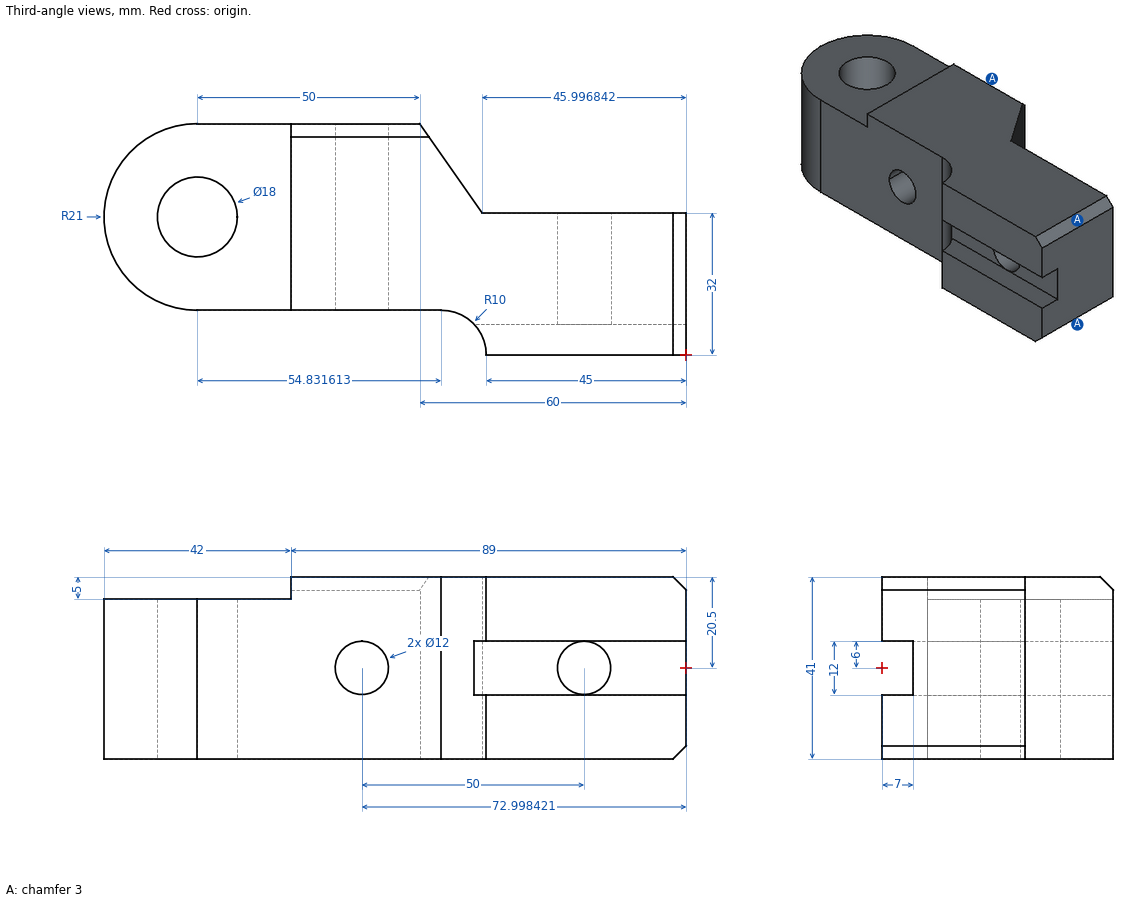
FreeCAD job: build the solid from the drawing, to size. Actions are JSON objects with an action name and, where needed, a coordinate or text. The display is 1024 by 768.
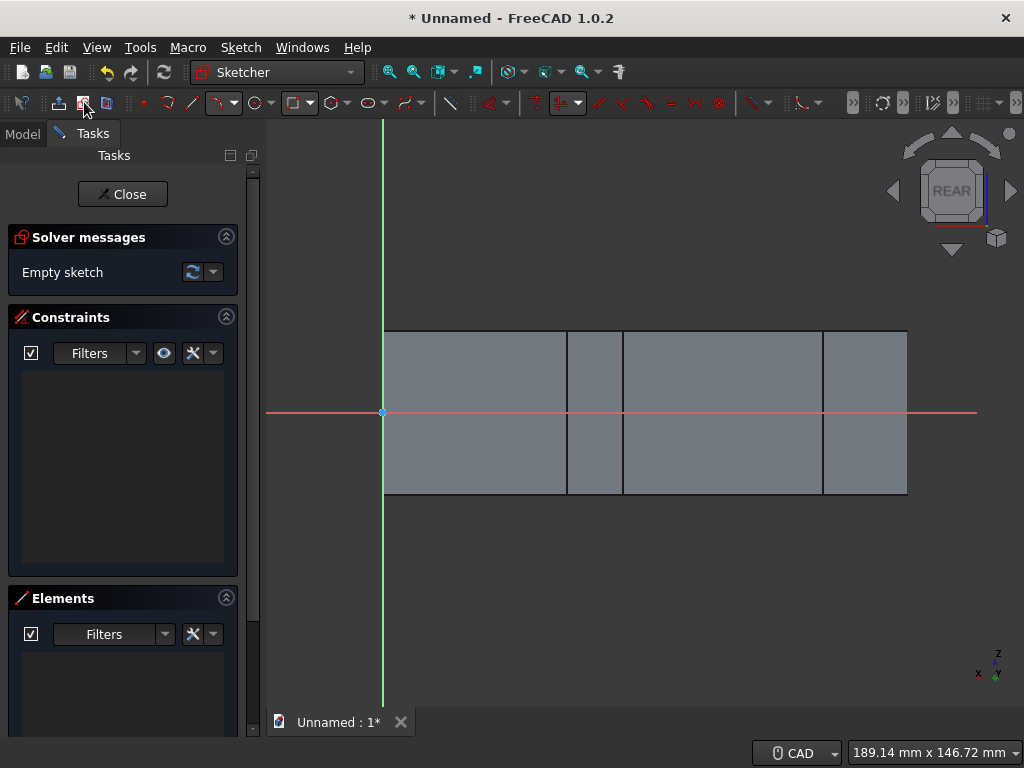
{"action": "scroll", "coordinate": [294, 544], "scroll_direction": "down", "scroll_amount": 1}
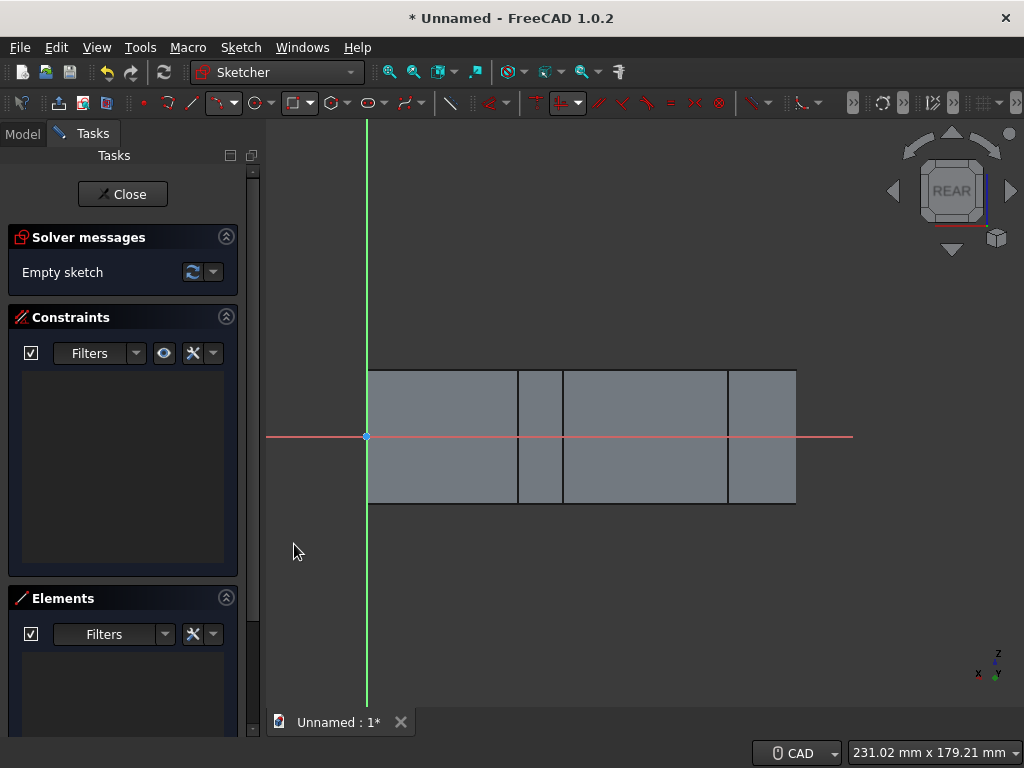
{"action": "left_click", "coordinate": [294, 104]}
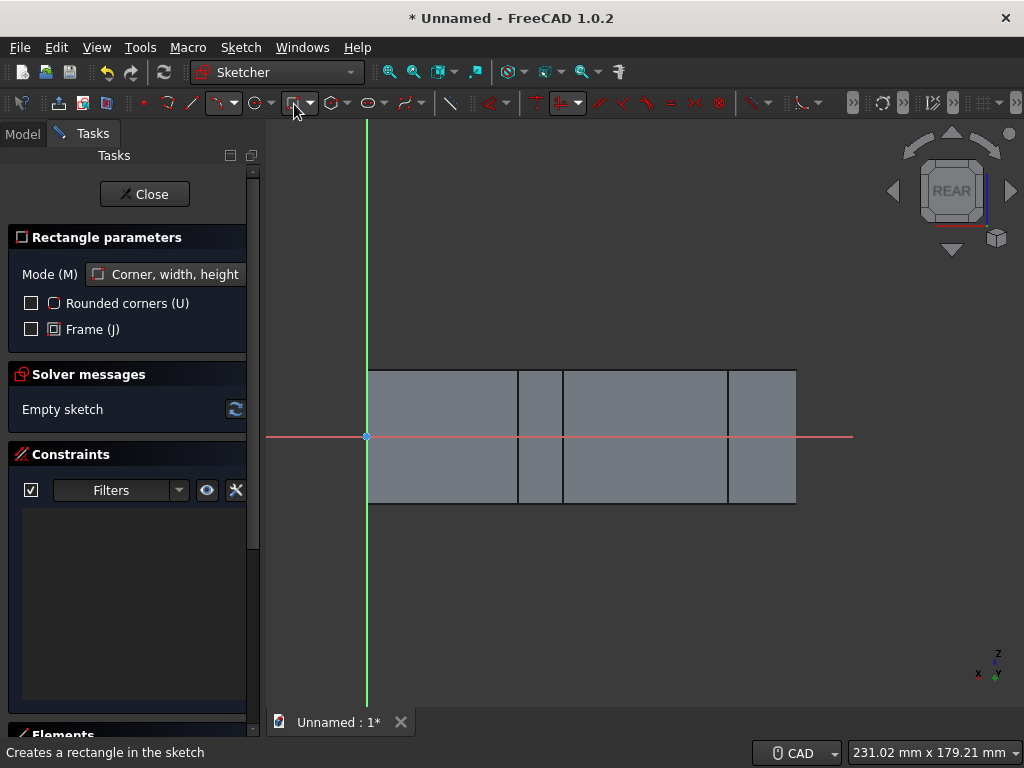
{"action": "left_click", "coordinate": [659, 370]}
{"action": "left_click", "coordinate": [796, 386]}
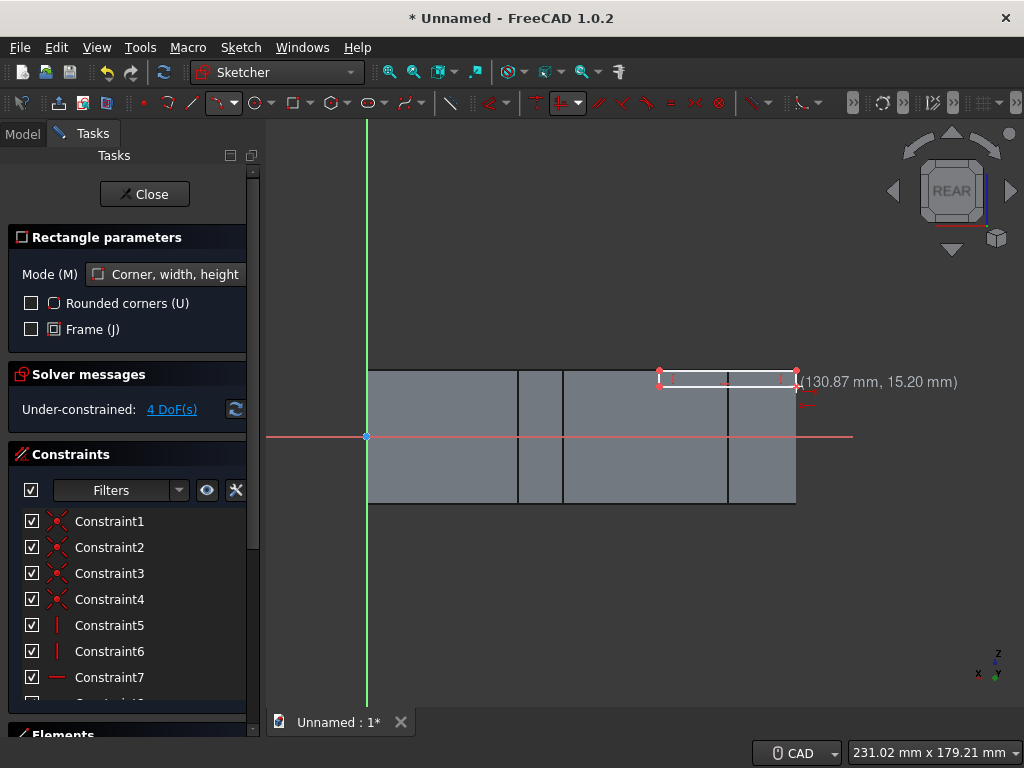
{"action": "left_click", "coordinate": [256, 104]}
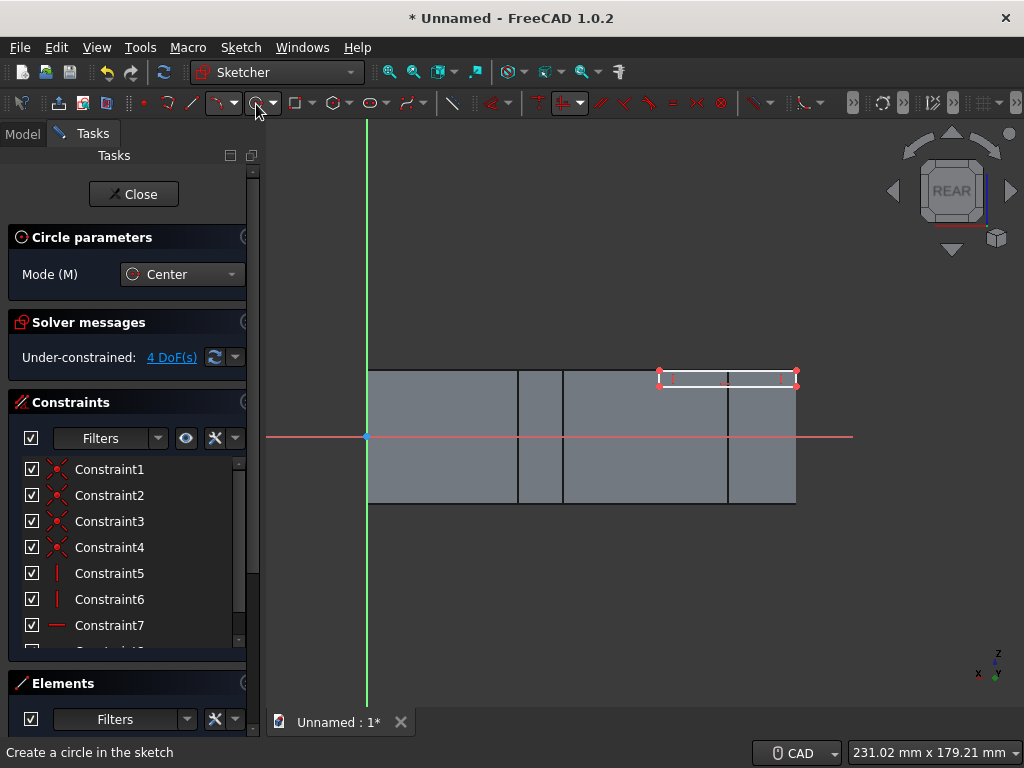
{"action": "left_click", "coordinate": [606, 437]}
{"action": "left_click", "coordinate": [613, 418]}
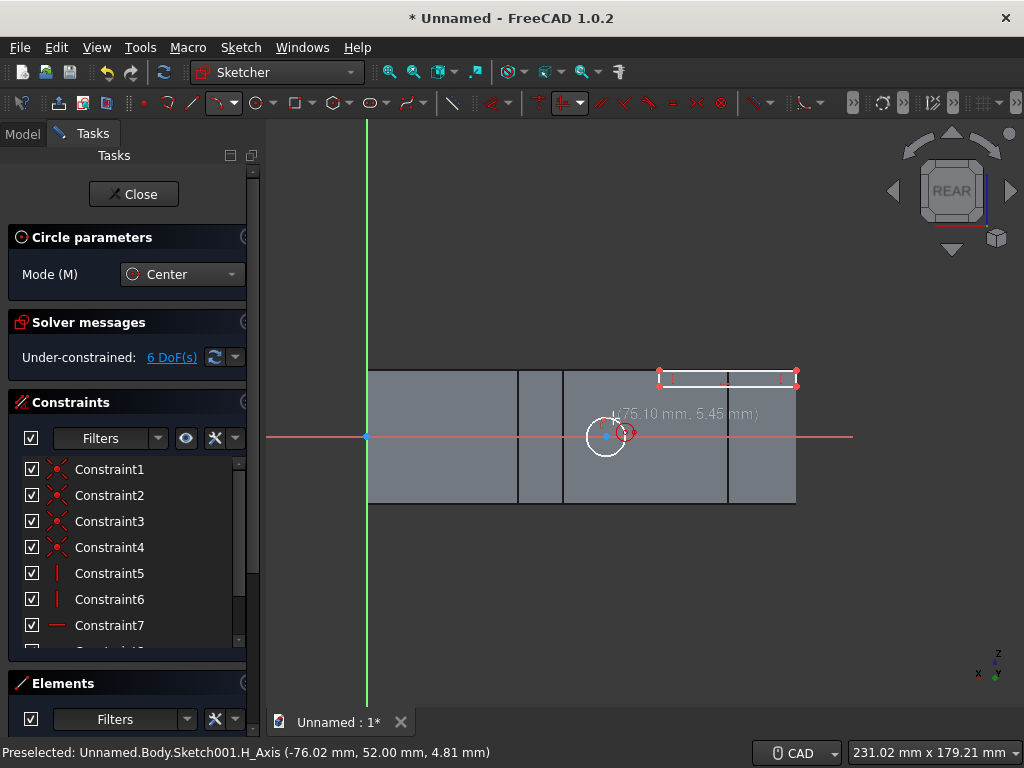
{"action": "left_click", "coordinate": [442, 437]}
{"action": "left_click", "coordinate": [449, 418]}
{"action": "key", "text": "Escape"}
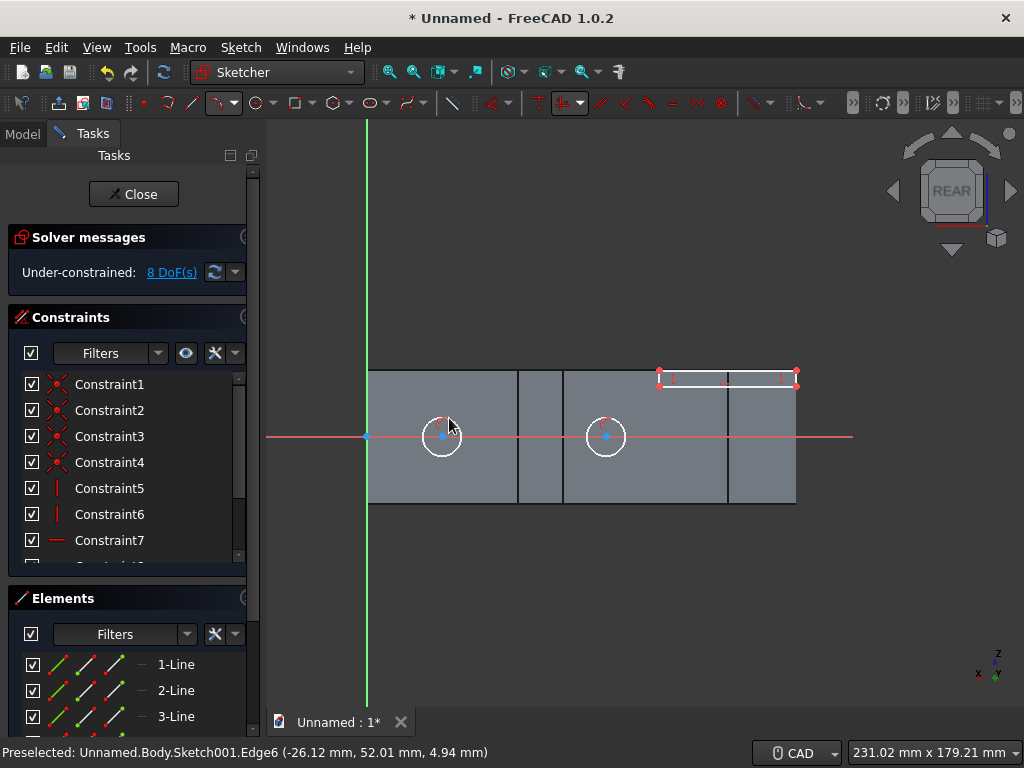
{"action": "left_click", "coordinate": [620, 423]}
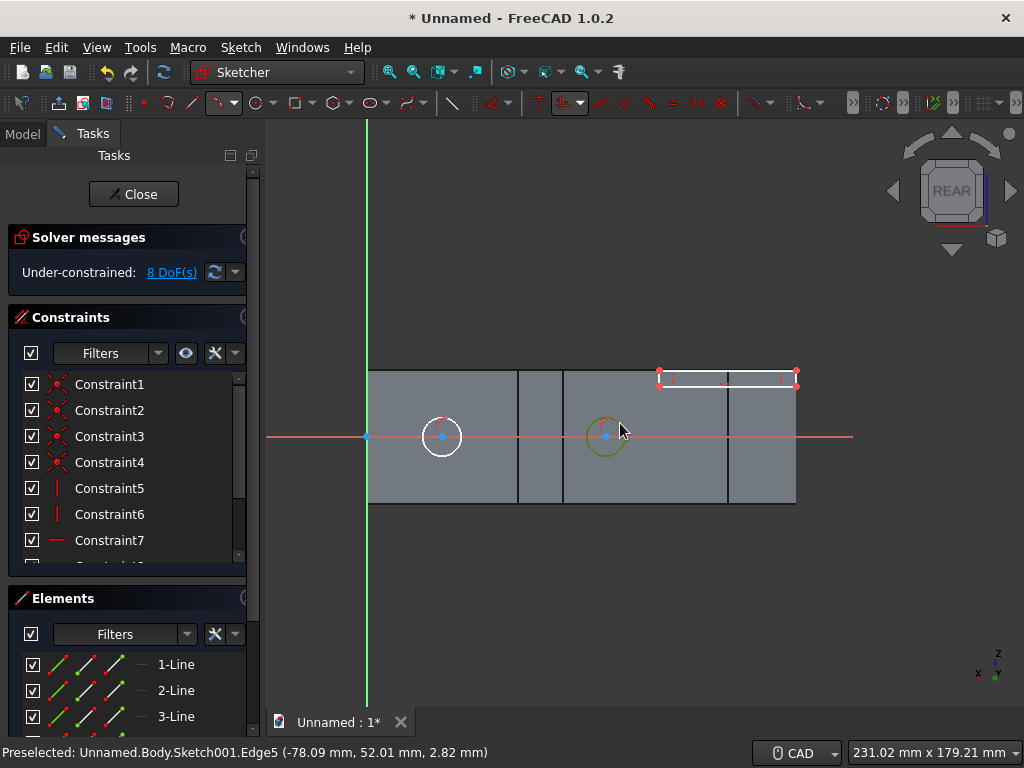
{"action": "left_click", "coordinate": [456, 423]}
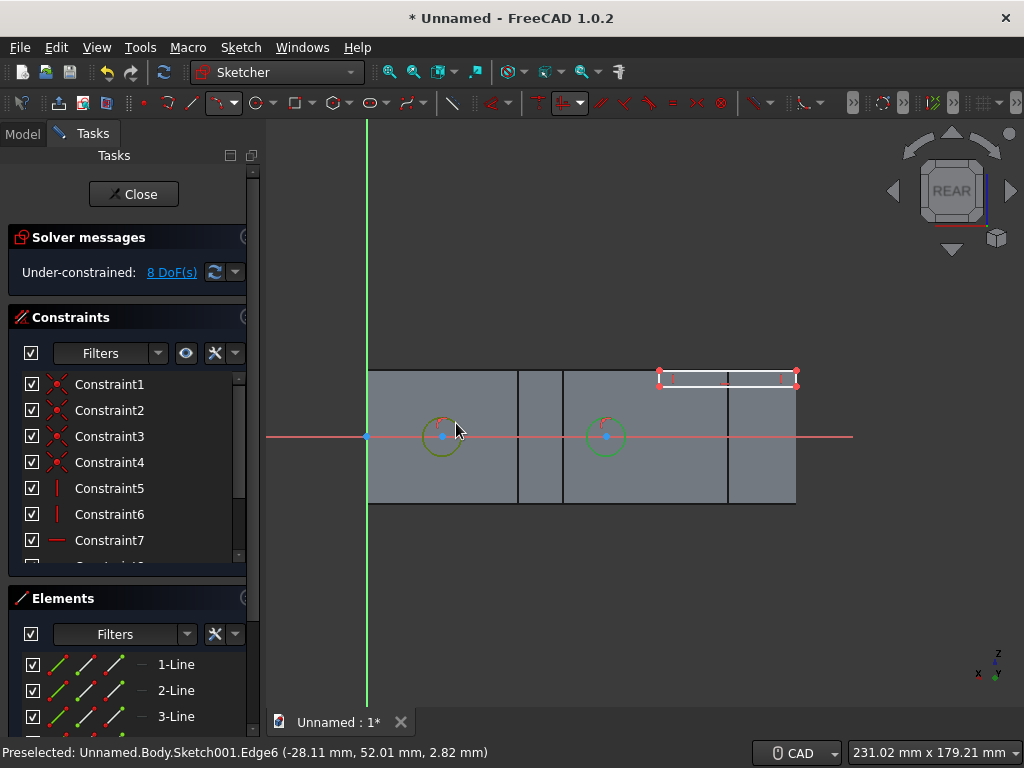
{"action": "left_click", "coordinate": [674, 104]}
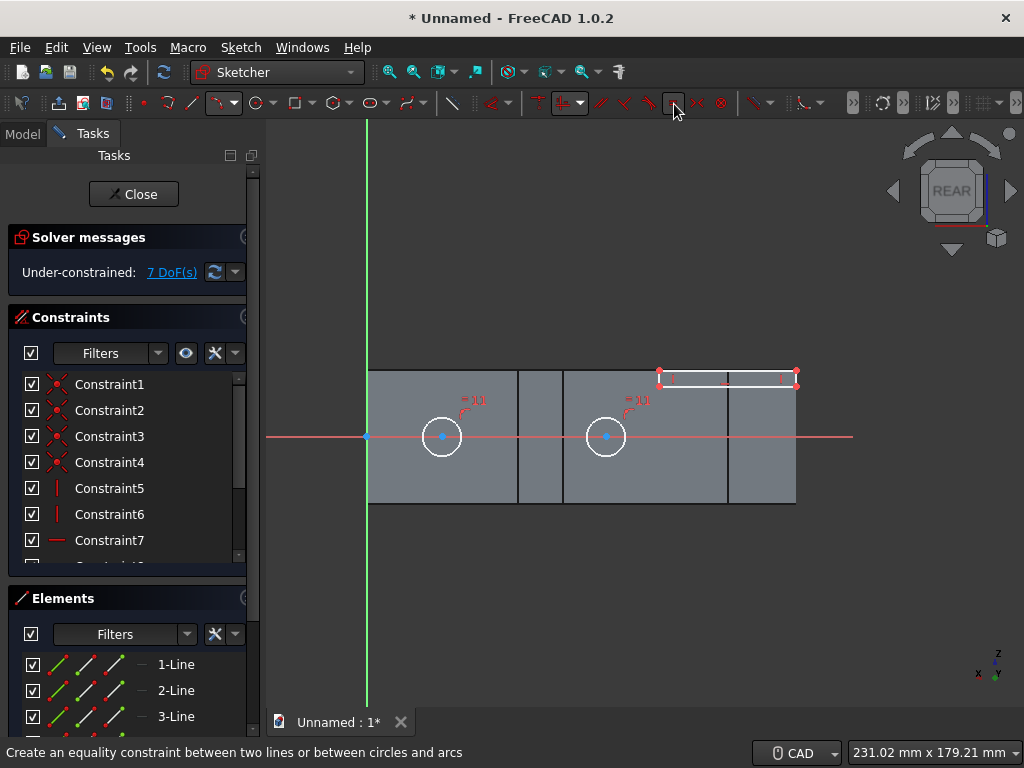
{"action": "left_click", "coordinate": [492, 104]}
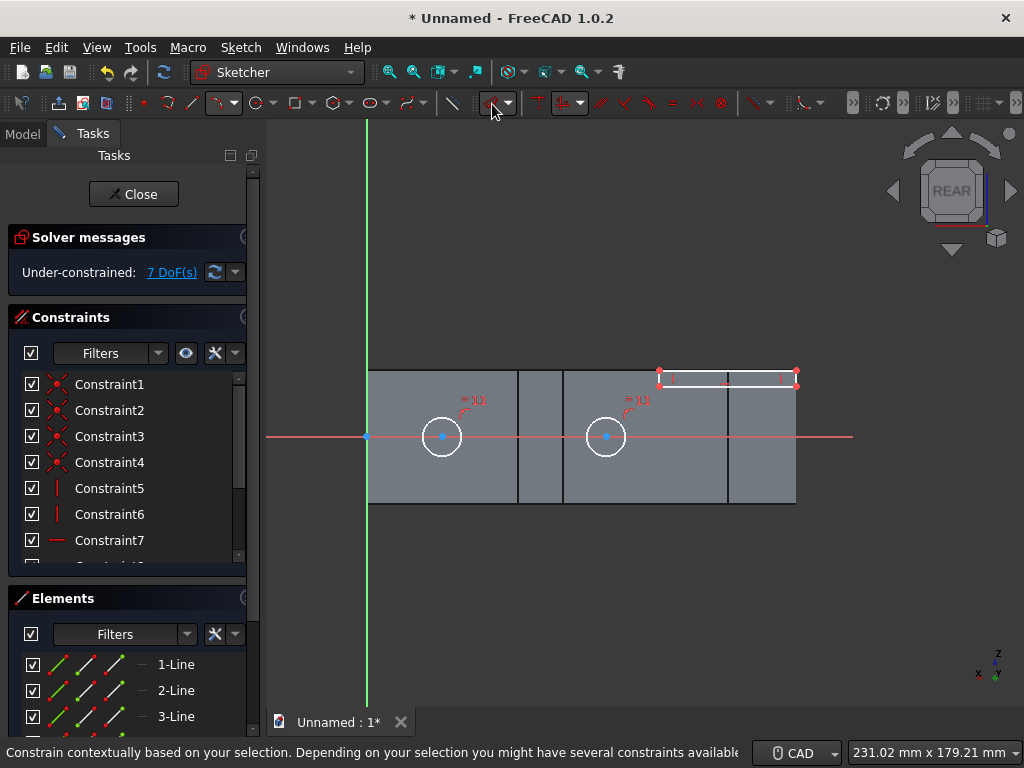
{"action": "left_click", "coordinate": [620, 423]}
{"action": "left_click", "coordinate": [643, 400]}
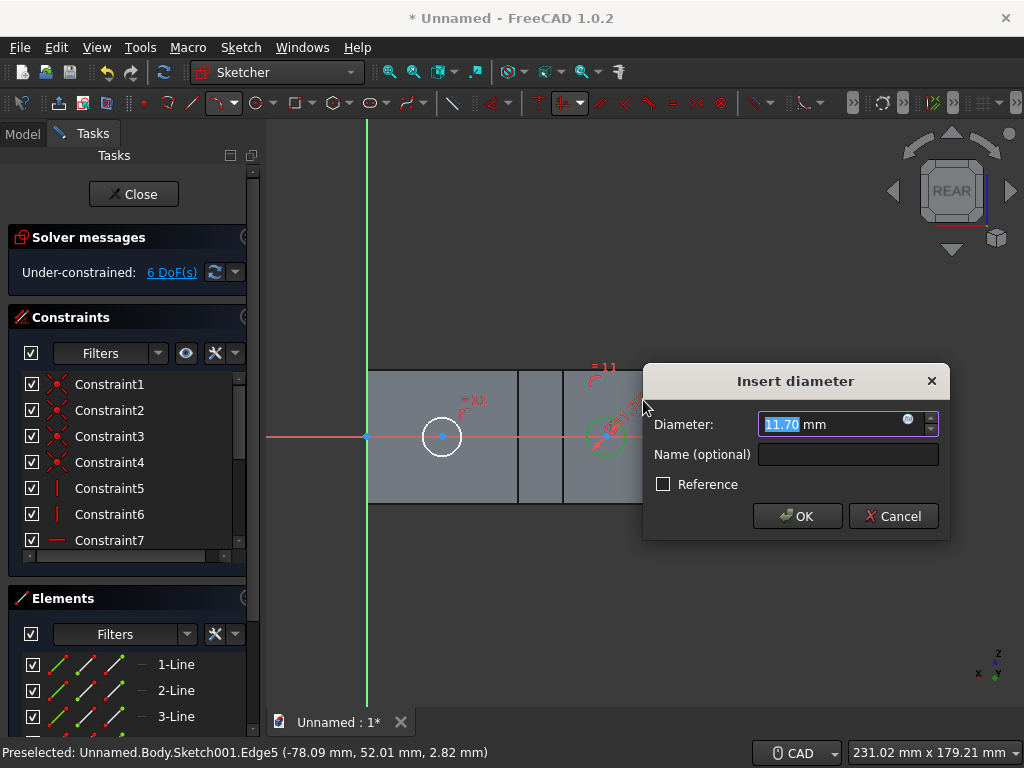
{"action": "type", "text": "12"}
{"action": "key", "text": "Return"}